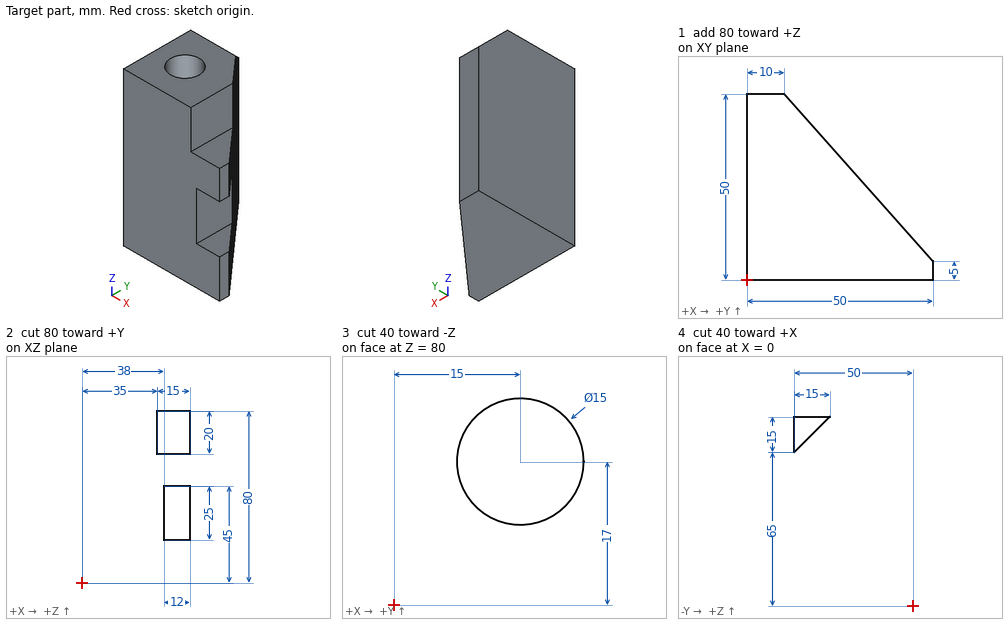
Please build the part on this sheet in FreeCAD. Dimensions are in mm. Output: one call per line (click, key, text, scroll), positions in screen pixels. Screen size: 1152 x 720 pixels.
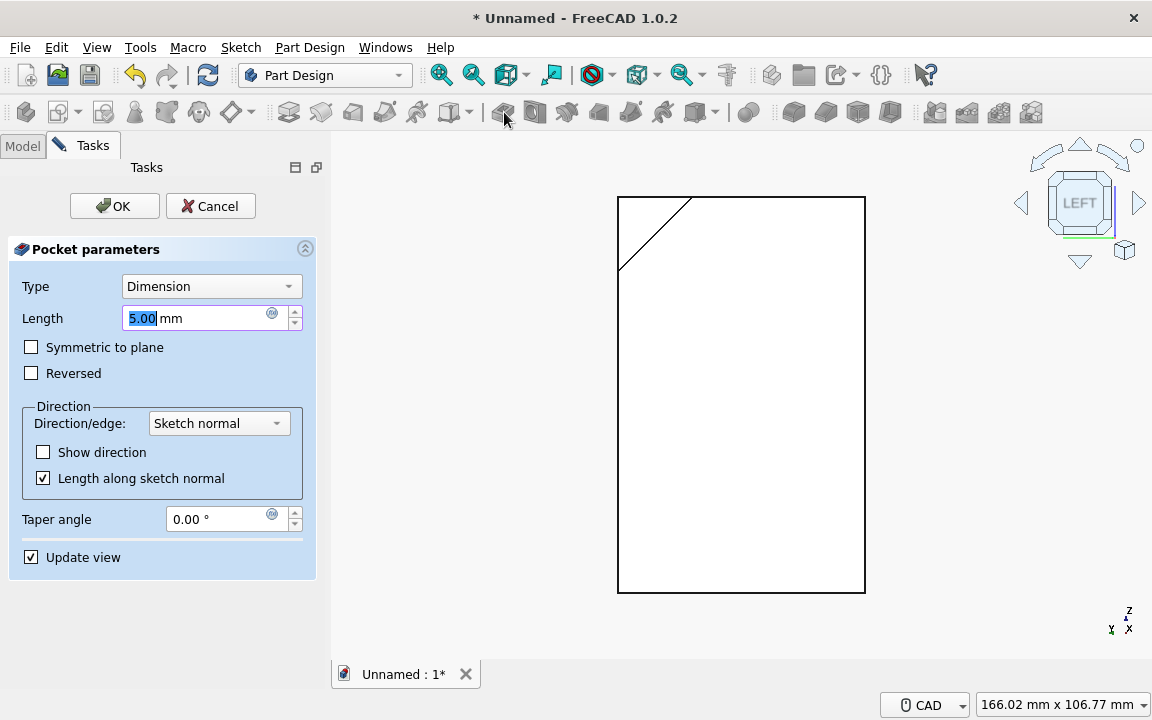
text(40)
key(Tab)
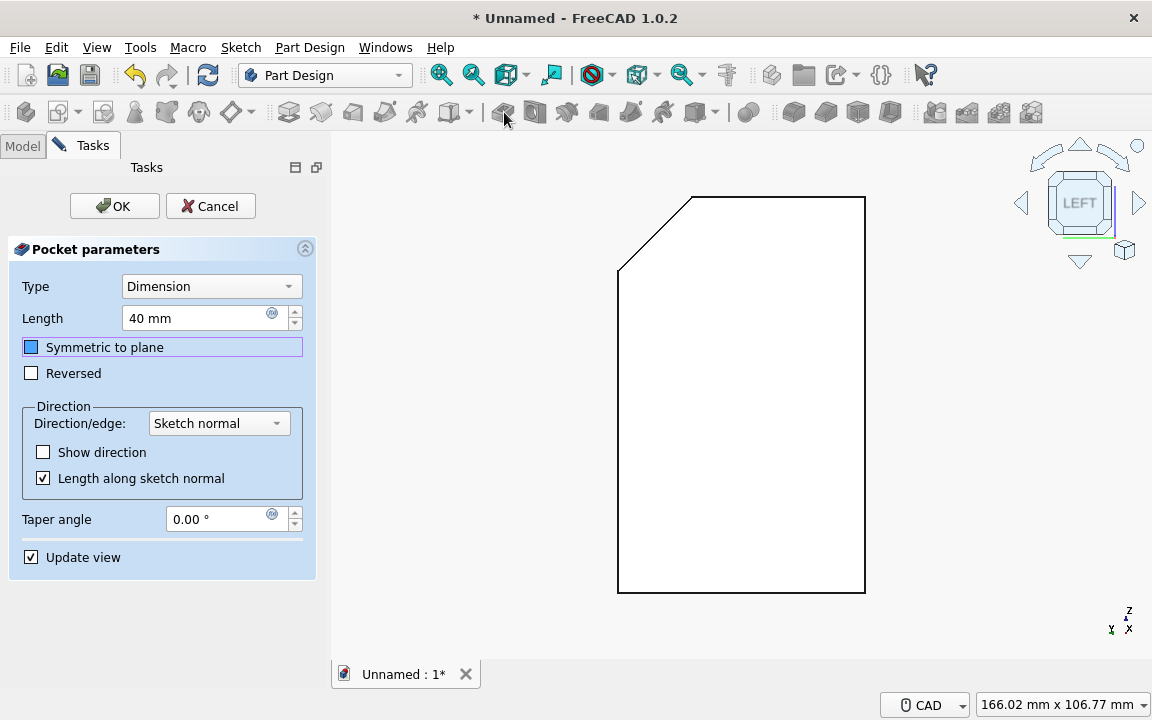
click(115, 206)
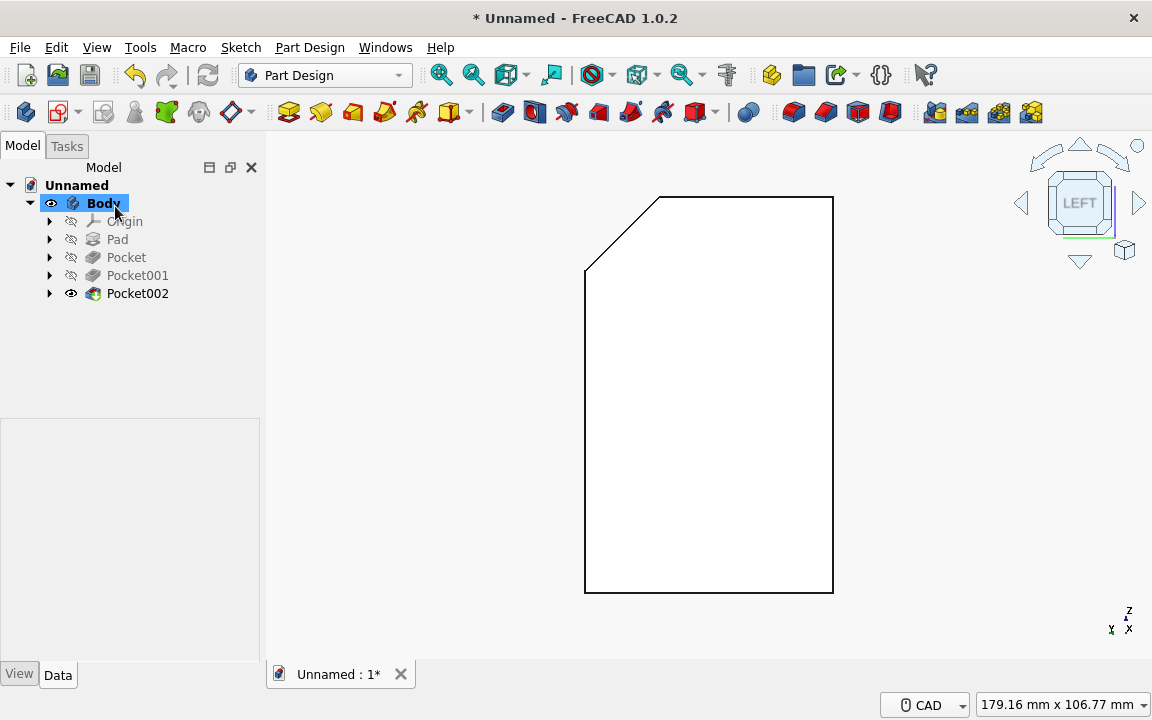
key(0)